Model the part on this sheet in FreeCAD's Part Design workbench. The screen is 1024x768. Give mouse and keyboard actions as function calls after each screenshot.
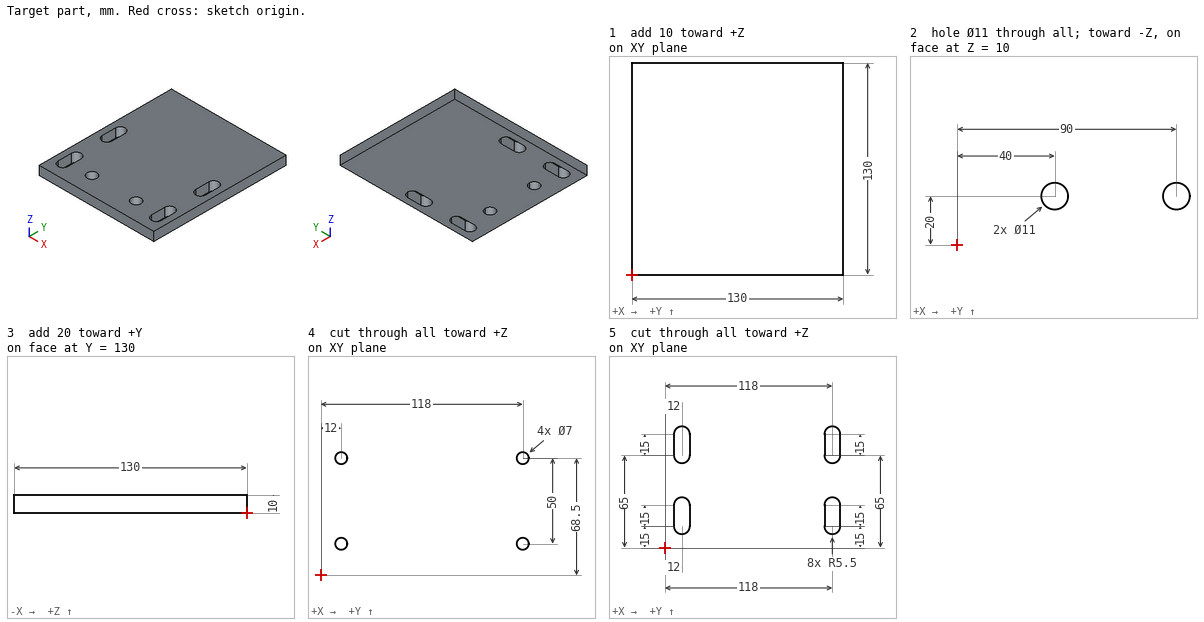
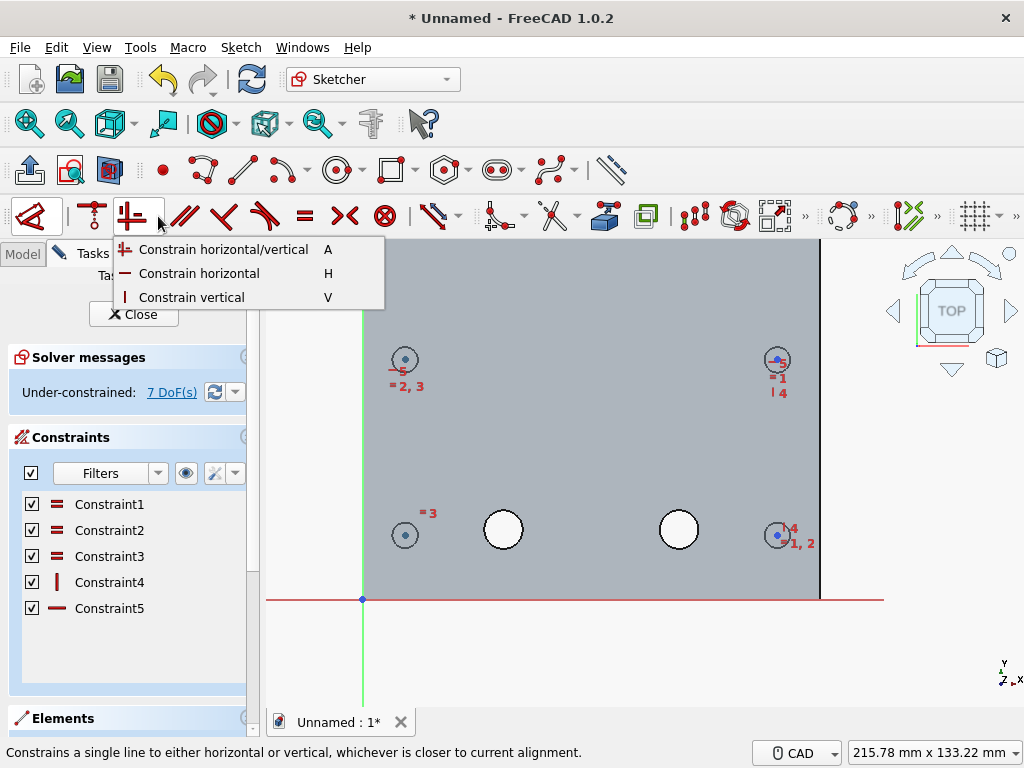
click(249, 297)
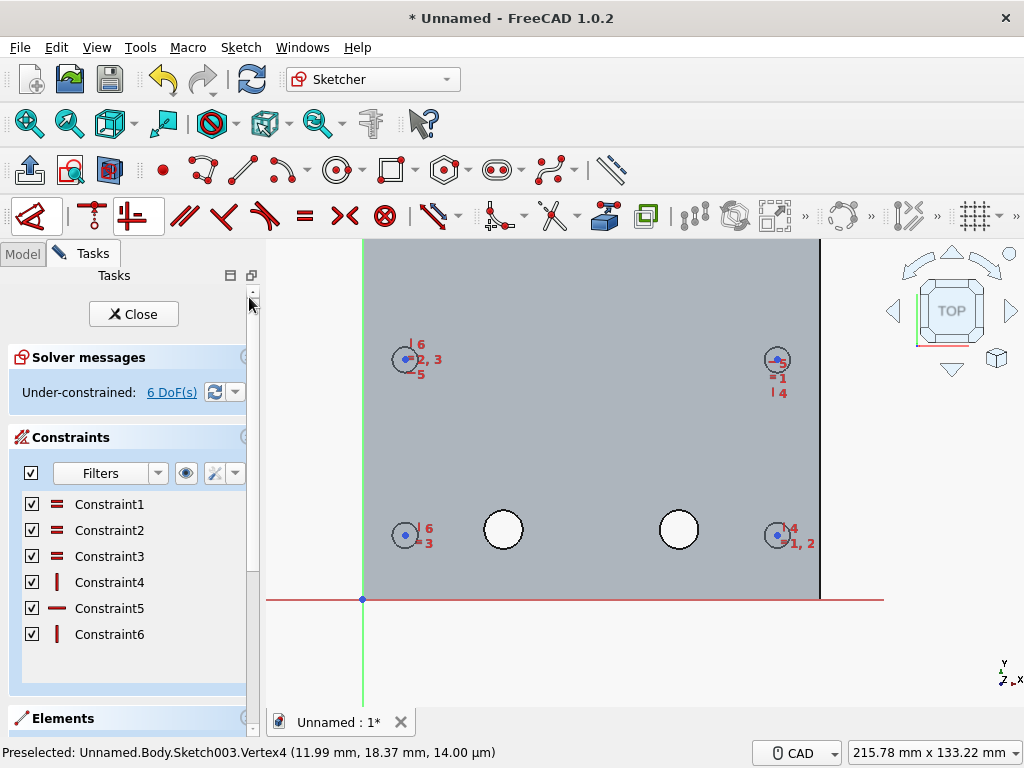
click(777, 535)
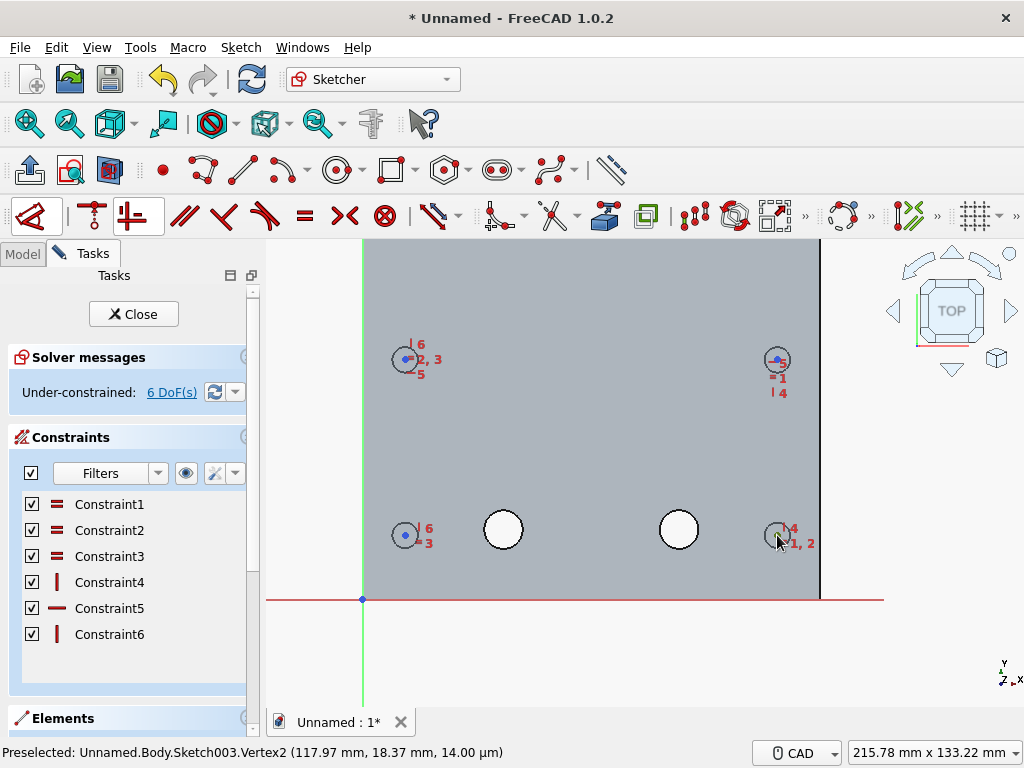
click(405, 535)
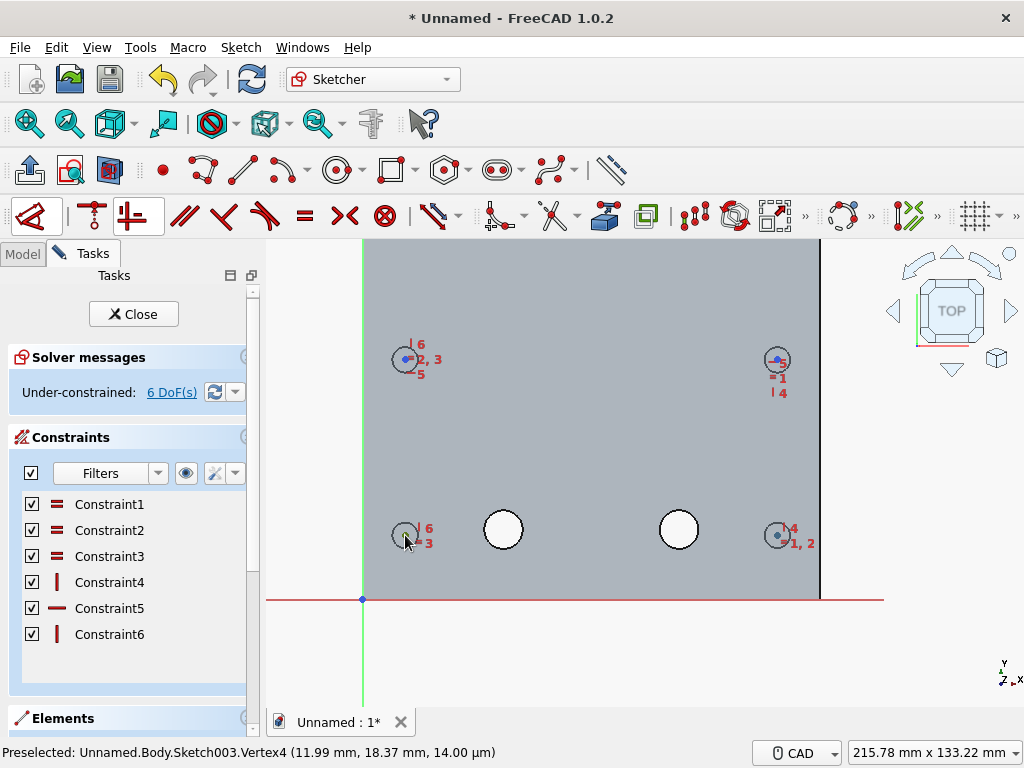
key(h)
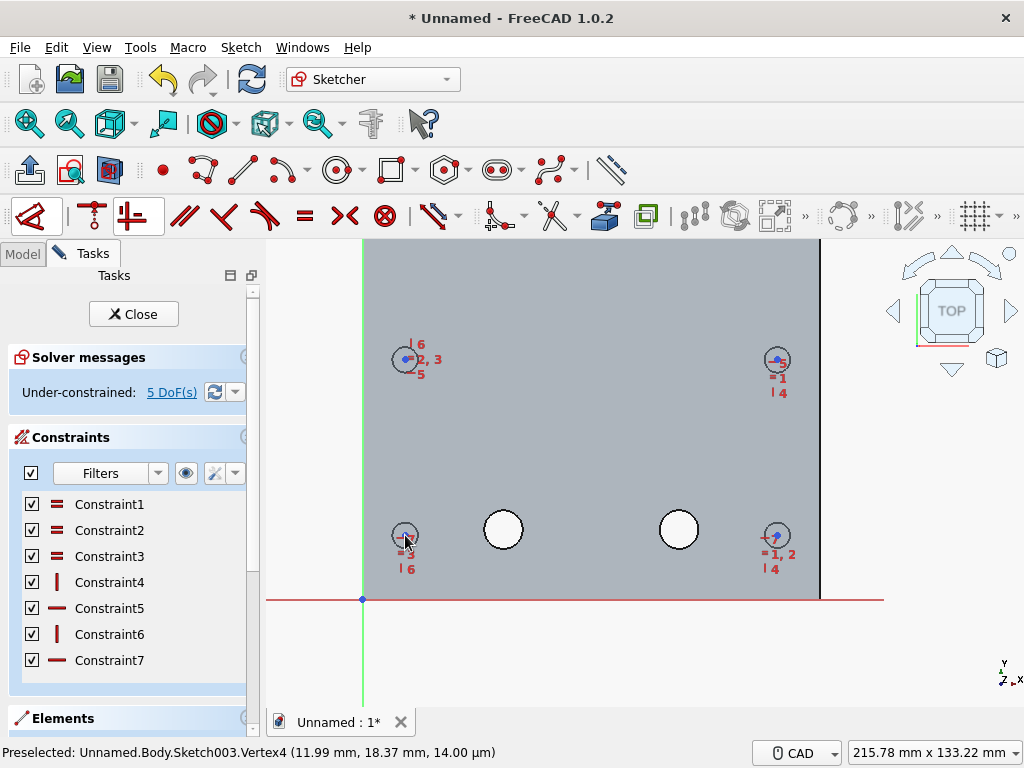
scroll(786, 351, up, 3)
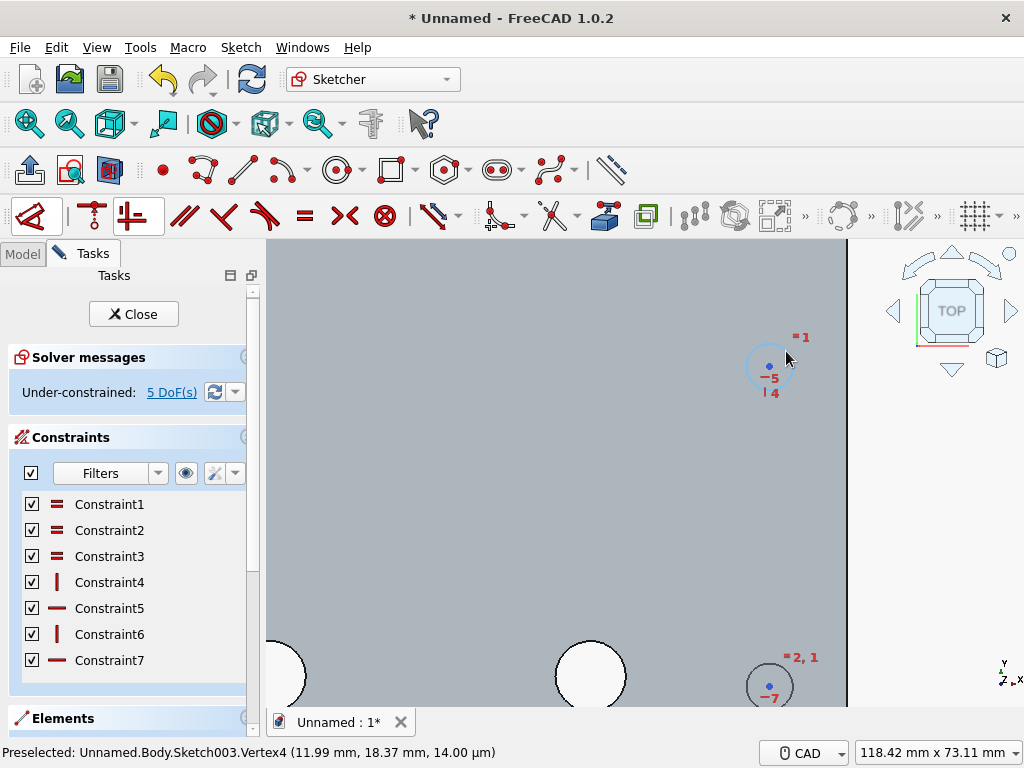
click(786, 351)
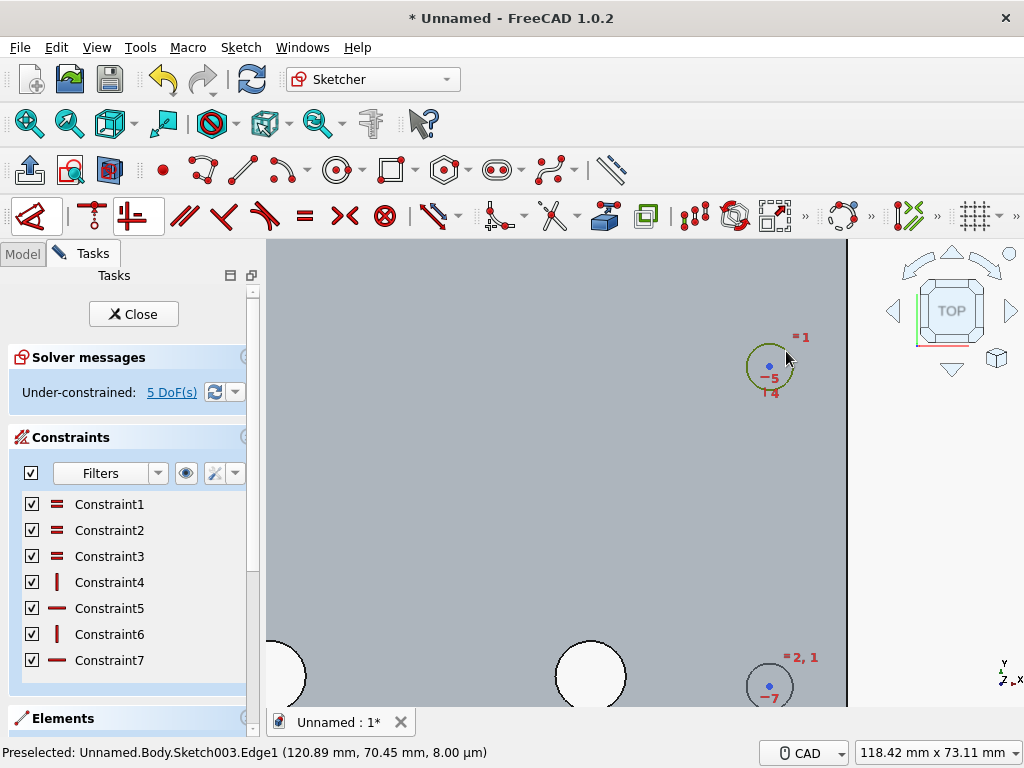
click(56, 216)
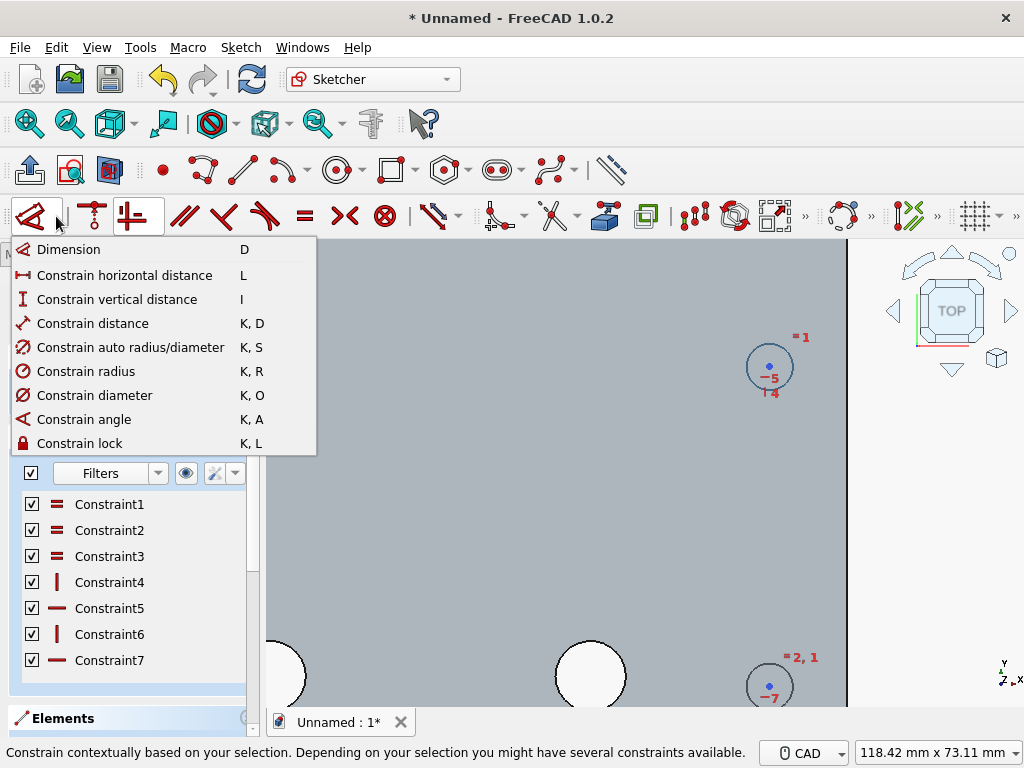
click(164, 395)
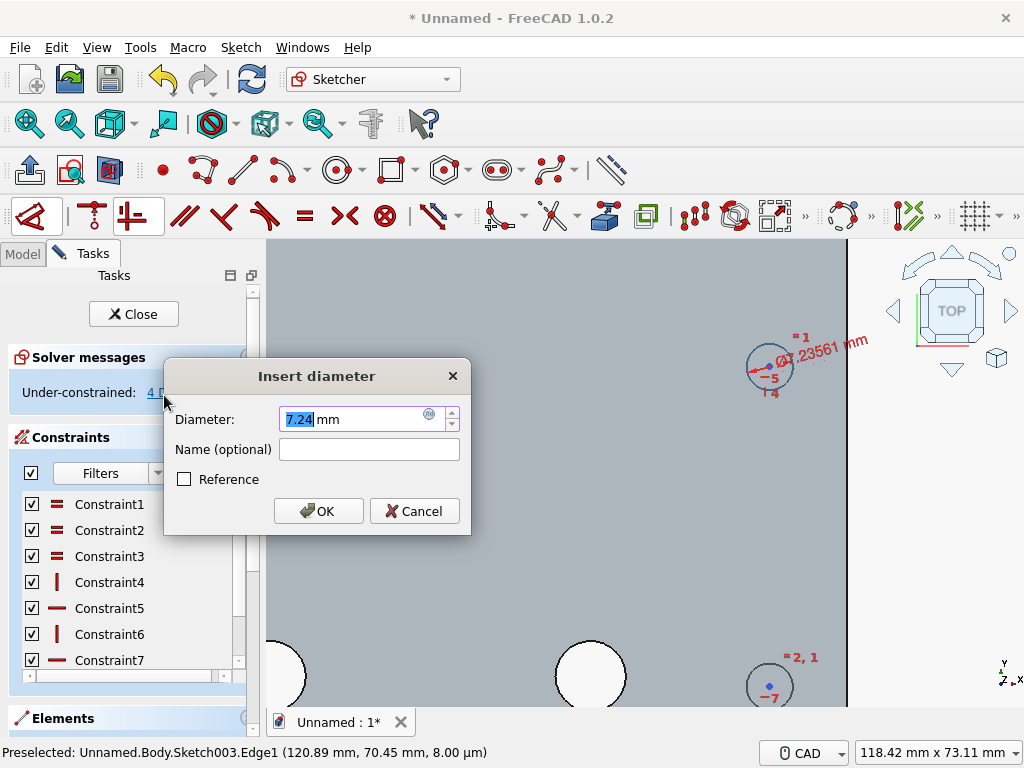
text(7)
key(Return)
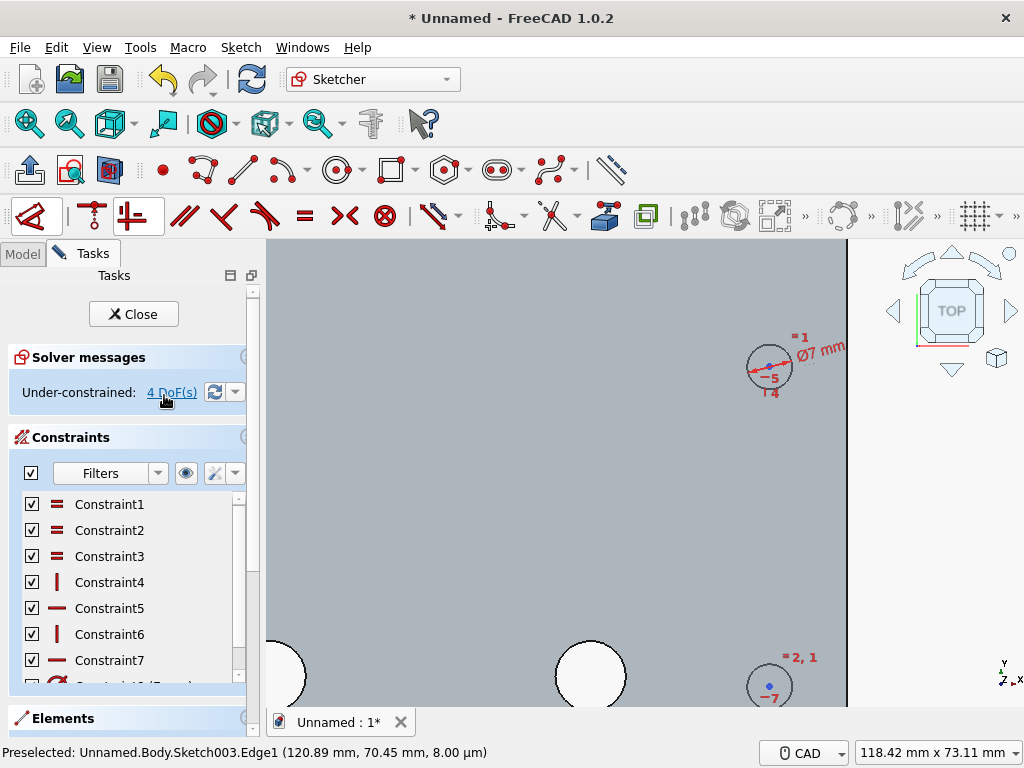
scroll(787, 350, down, 3)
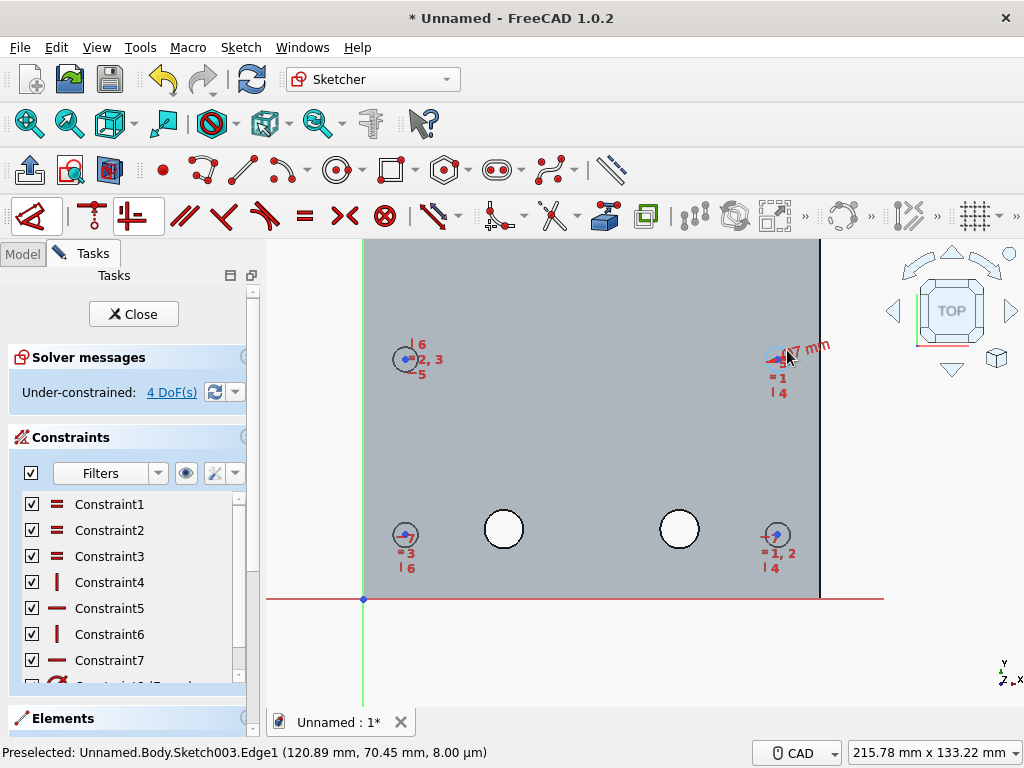
click(406, 359)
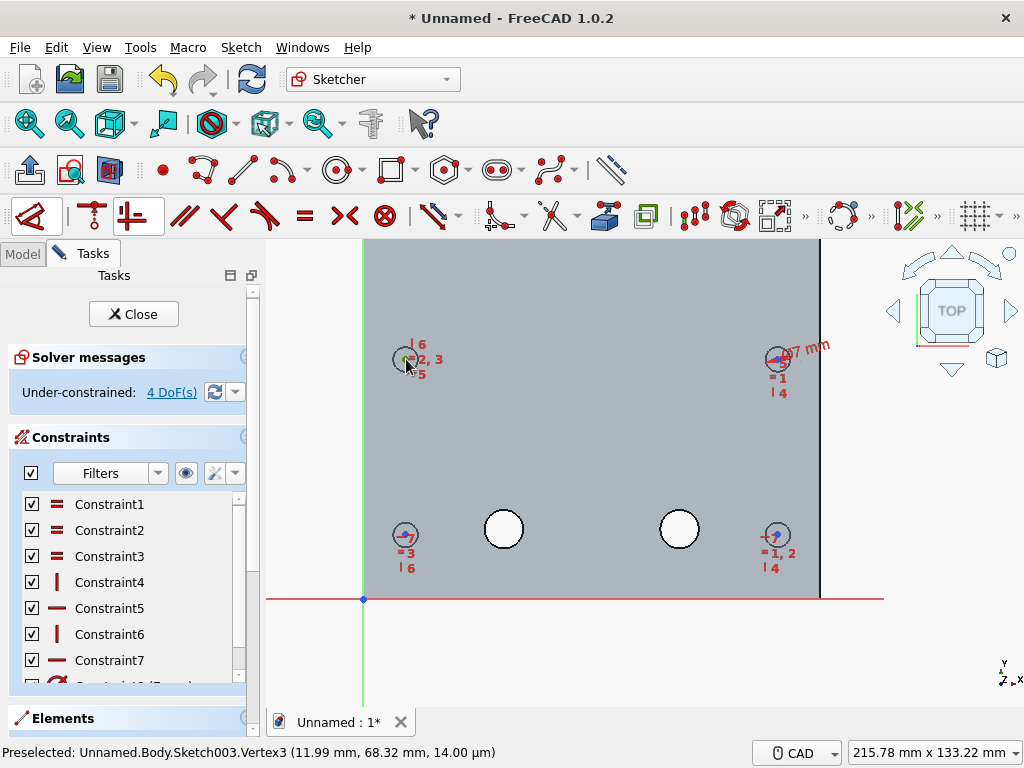
key(l)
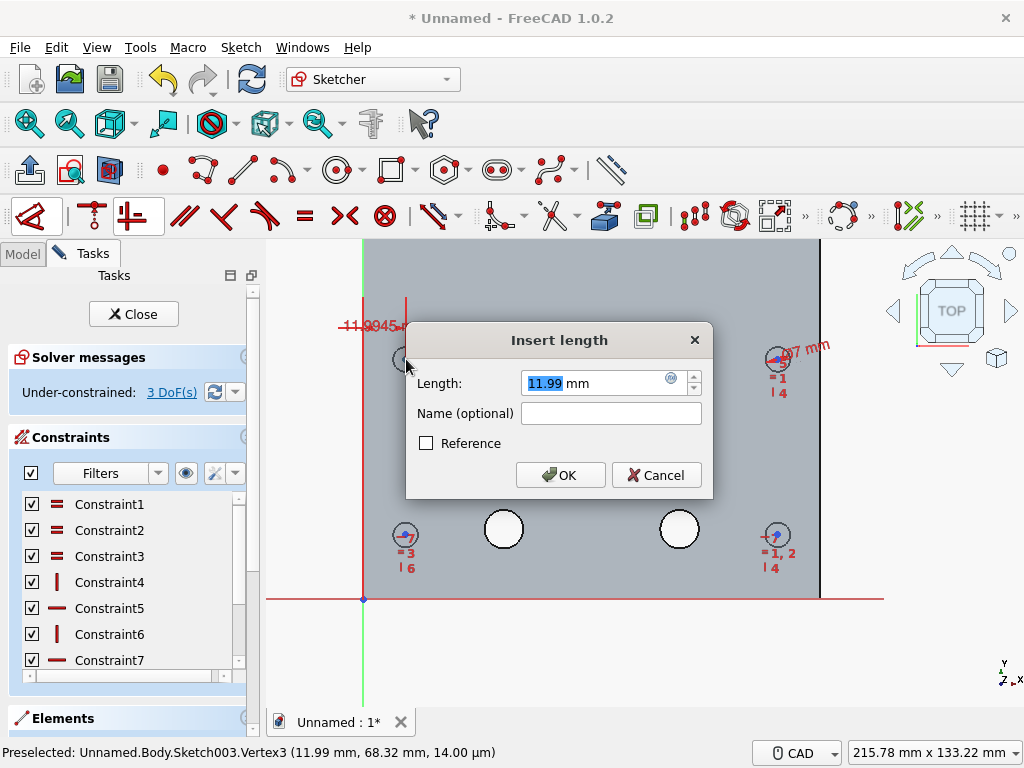
text(12)
key(Return)